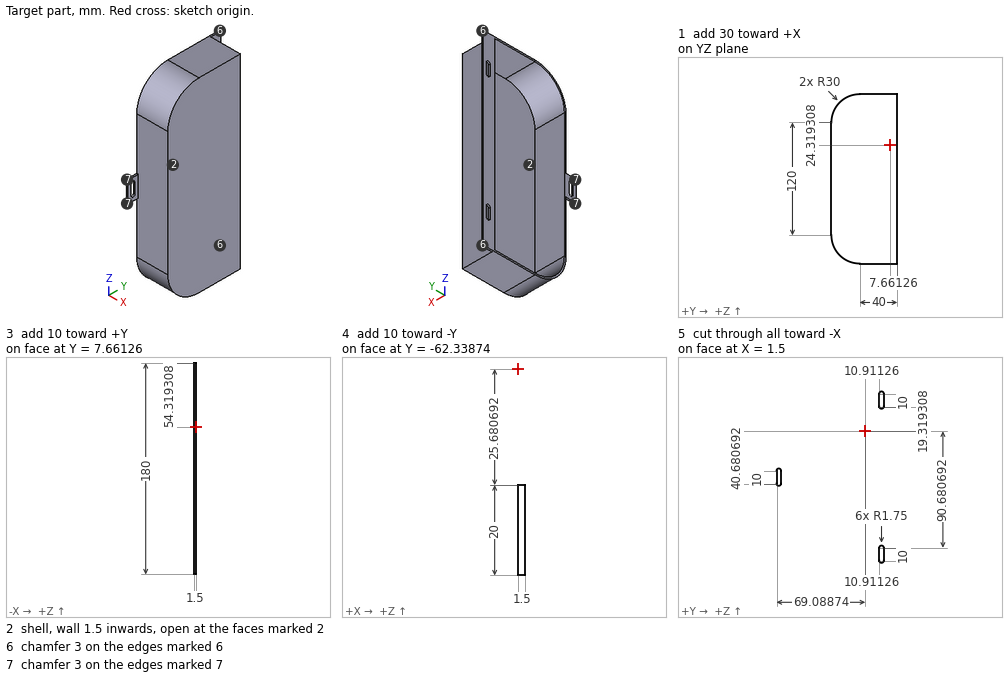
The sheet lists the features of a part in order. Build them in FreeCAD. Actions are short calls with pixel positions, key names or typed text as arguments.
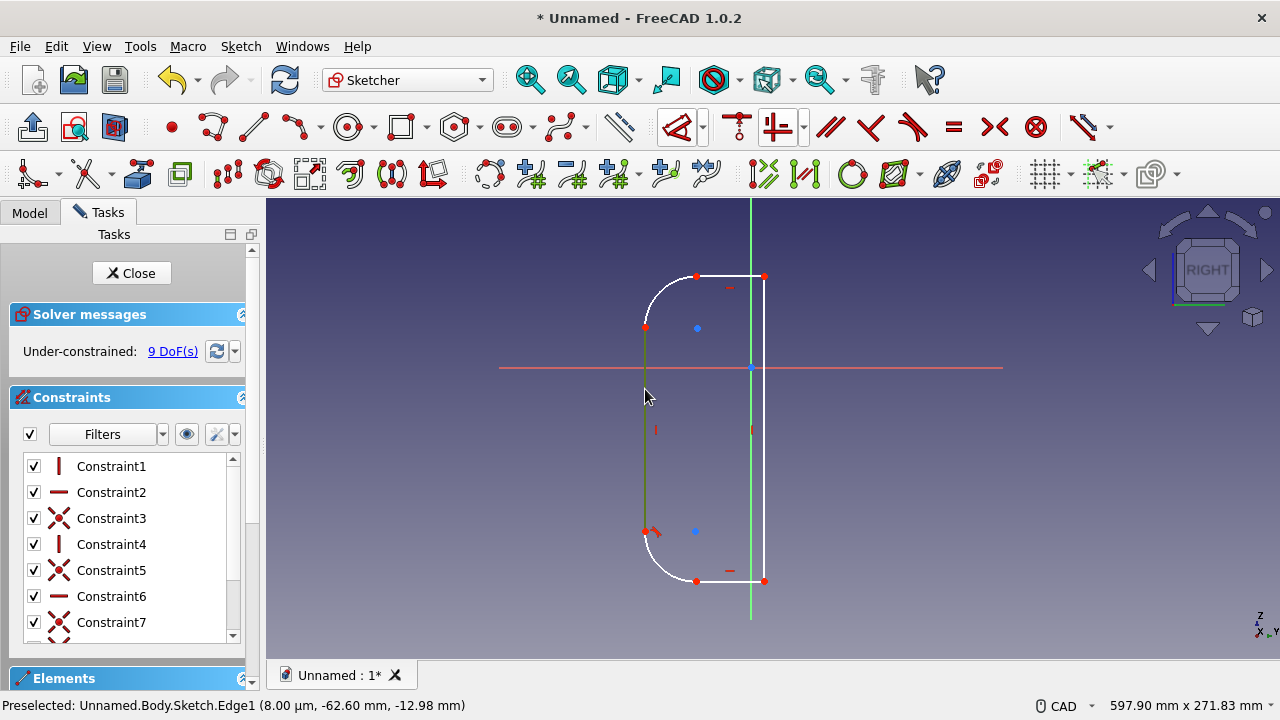
click(673, 282)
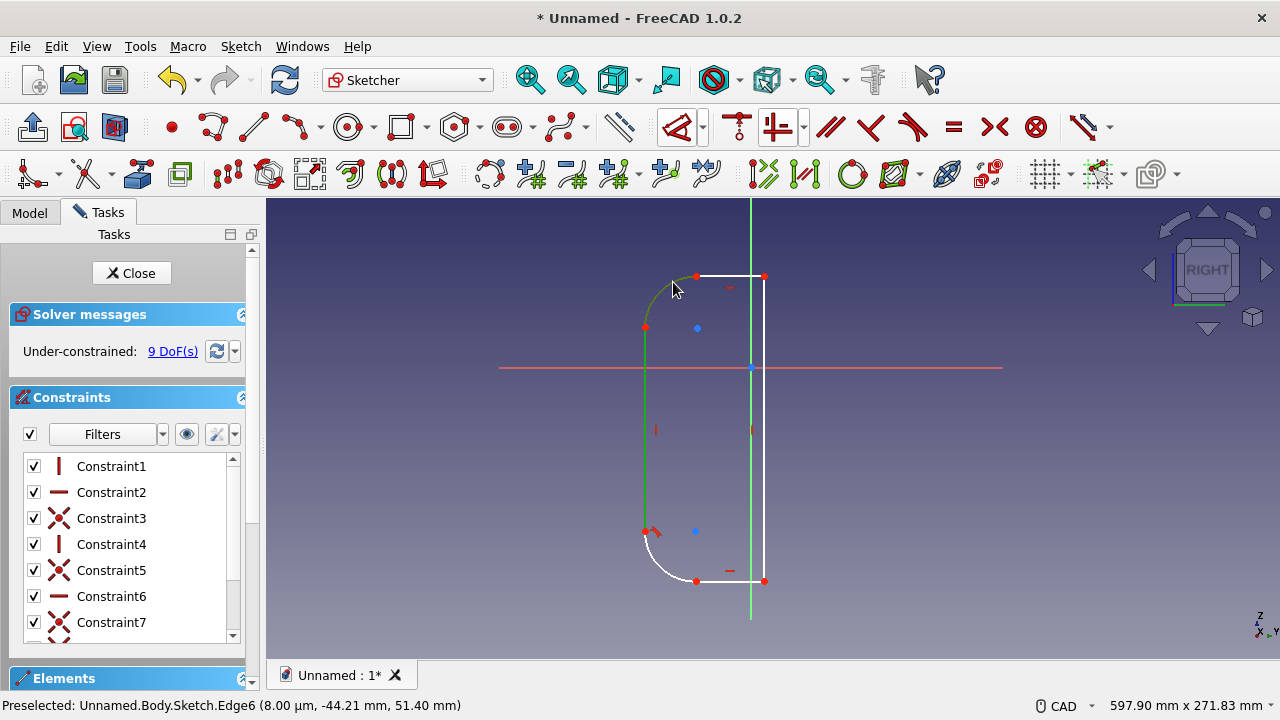
click(913, 128)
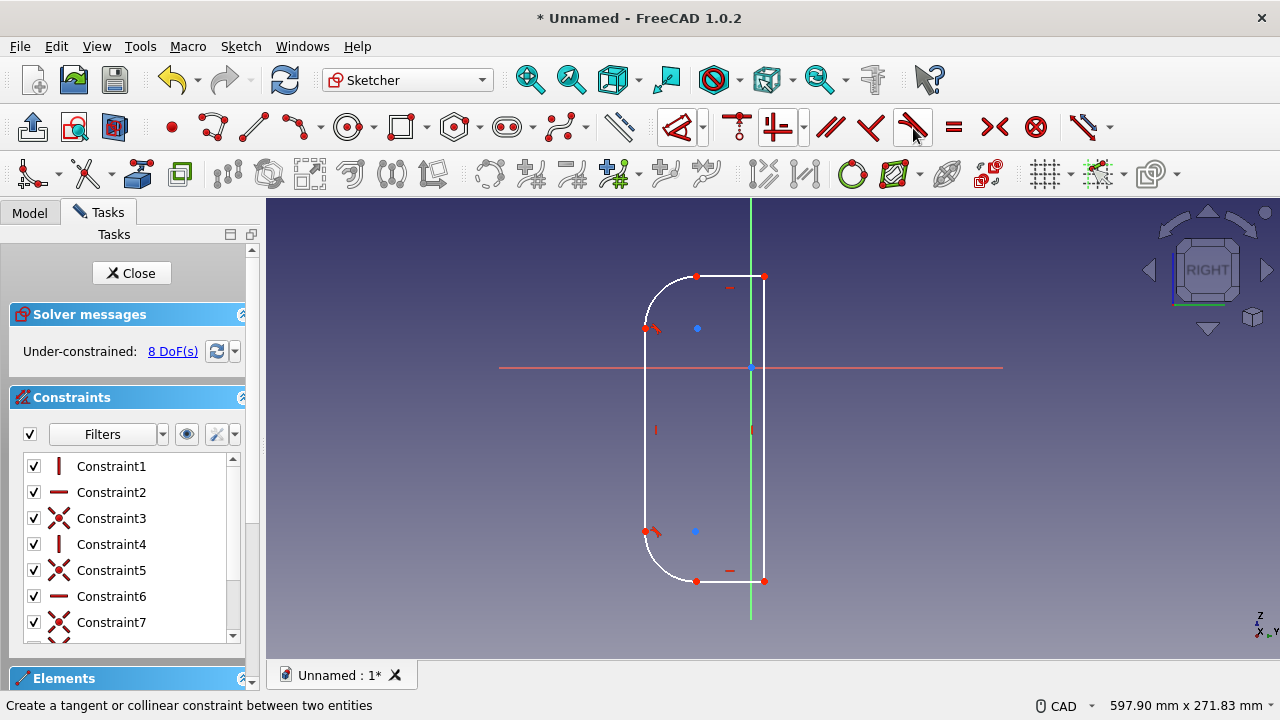
click(716, 582)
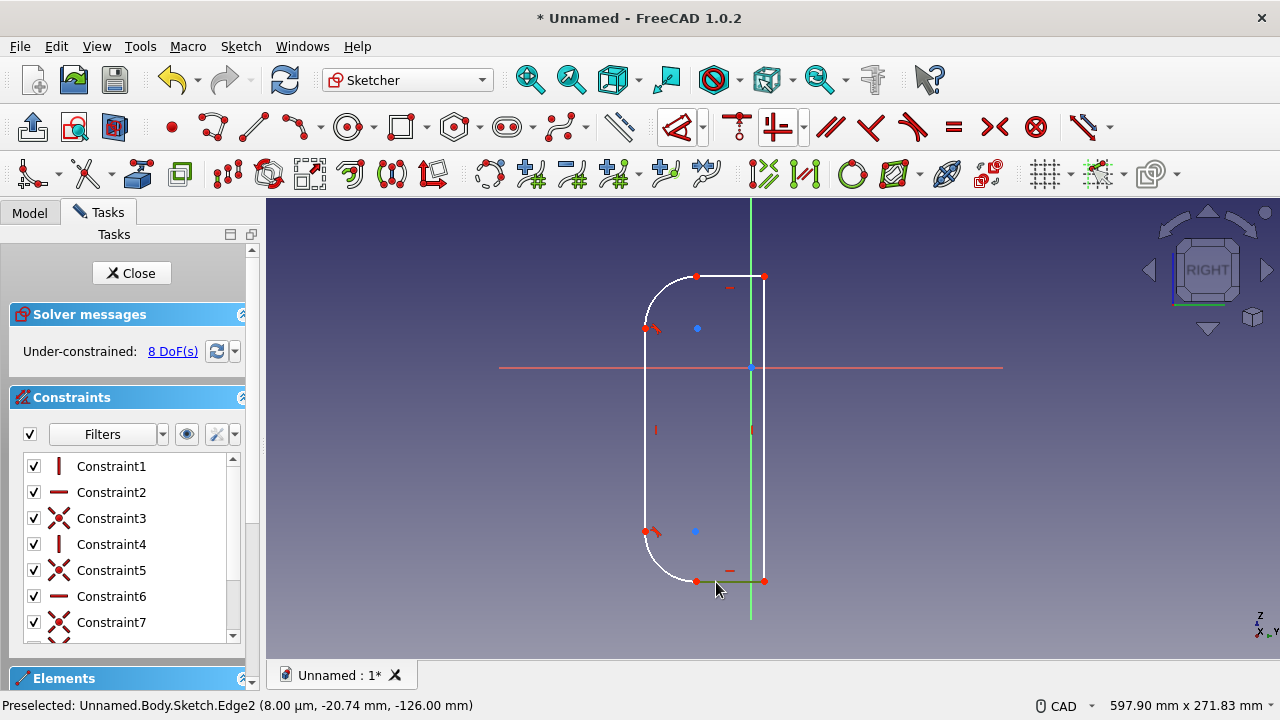
click(651, 554)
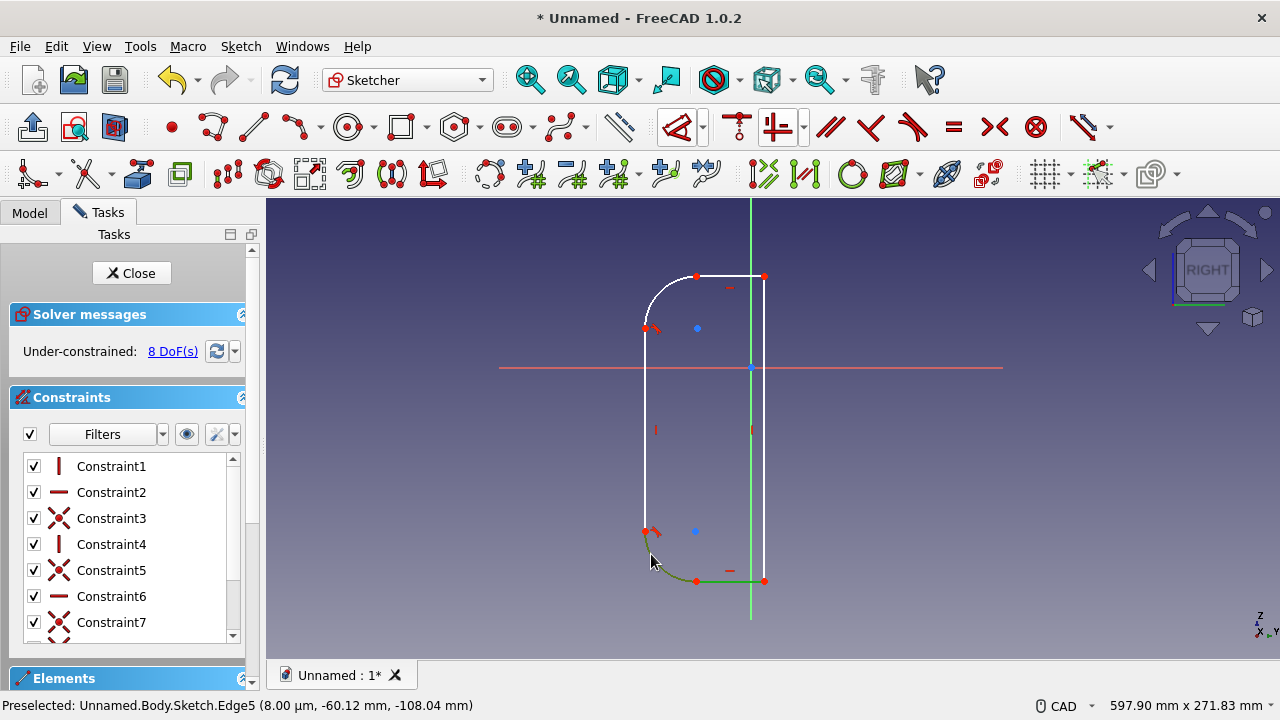
click(913, 128)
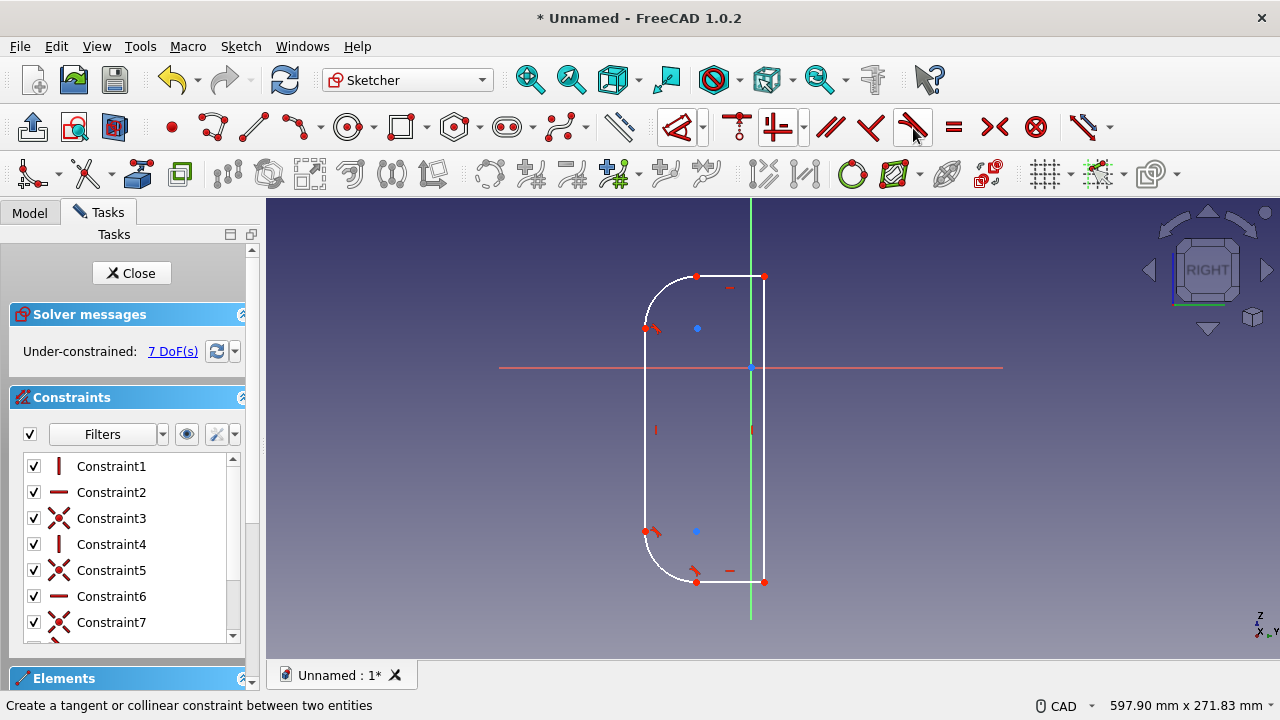
click(717, 276)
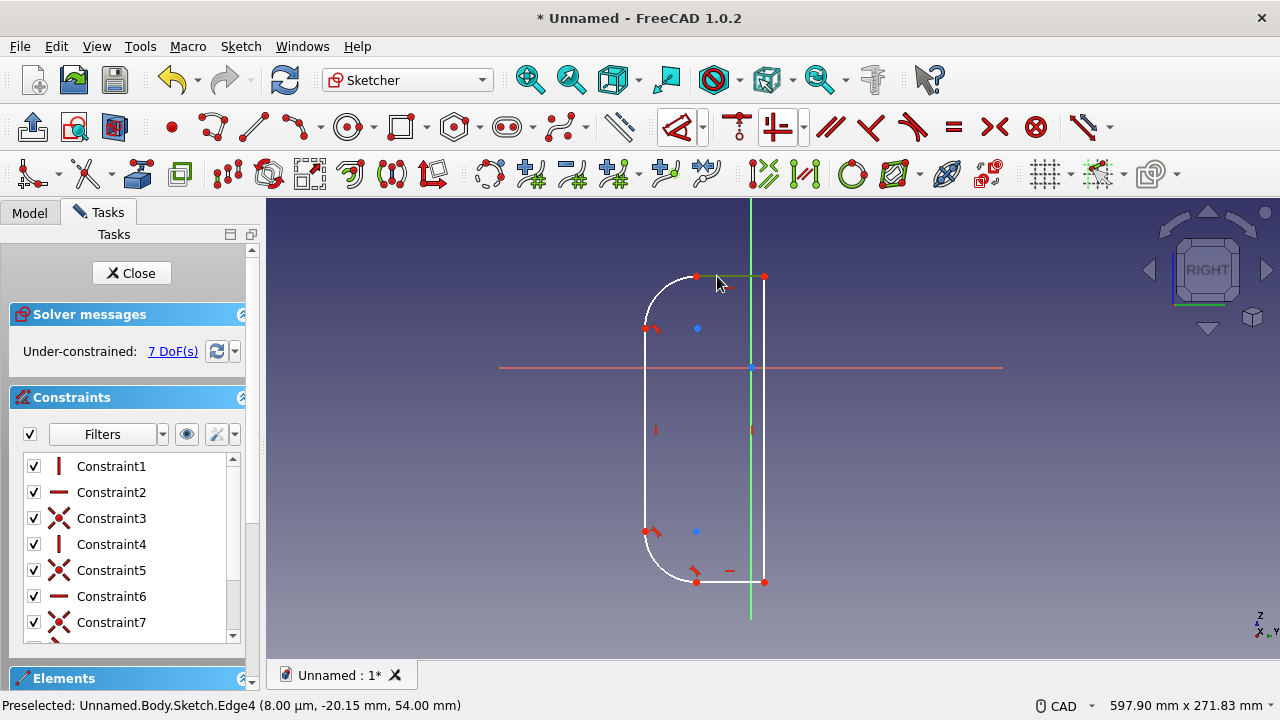
click(673, 282)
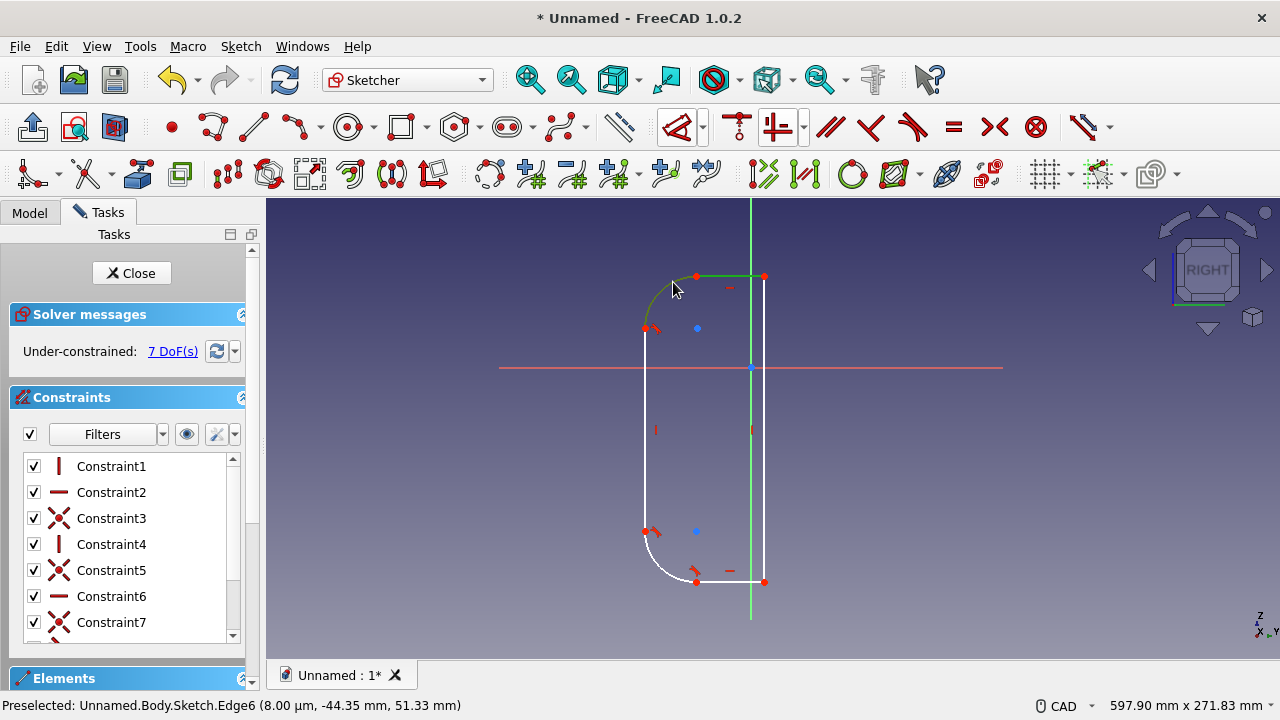
click(913, 128)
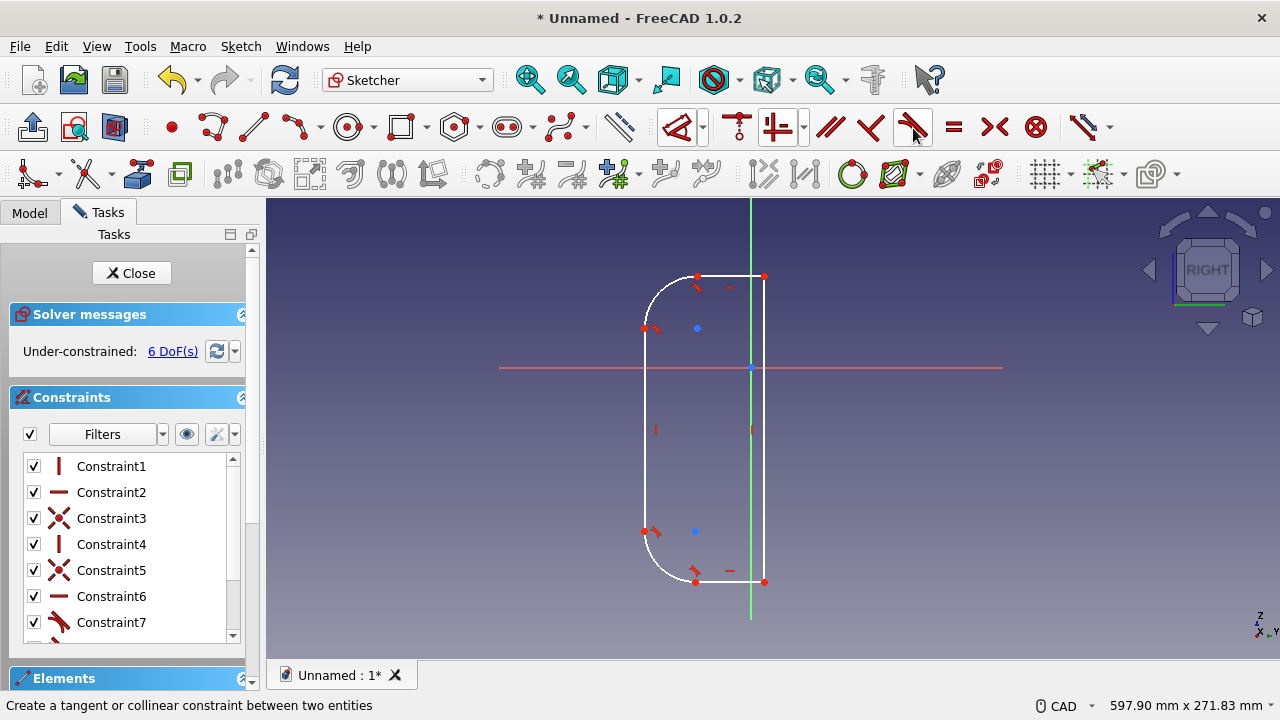
click(650, 554)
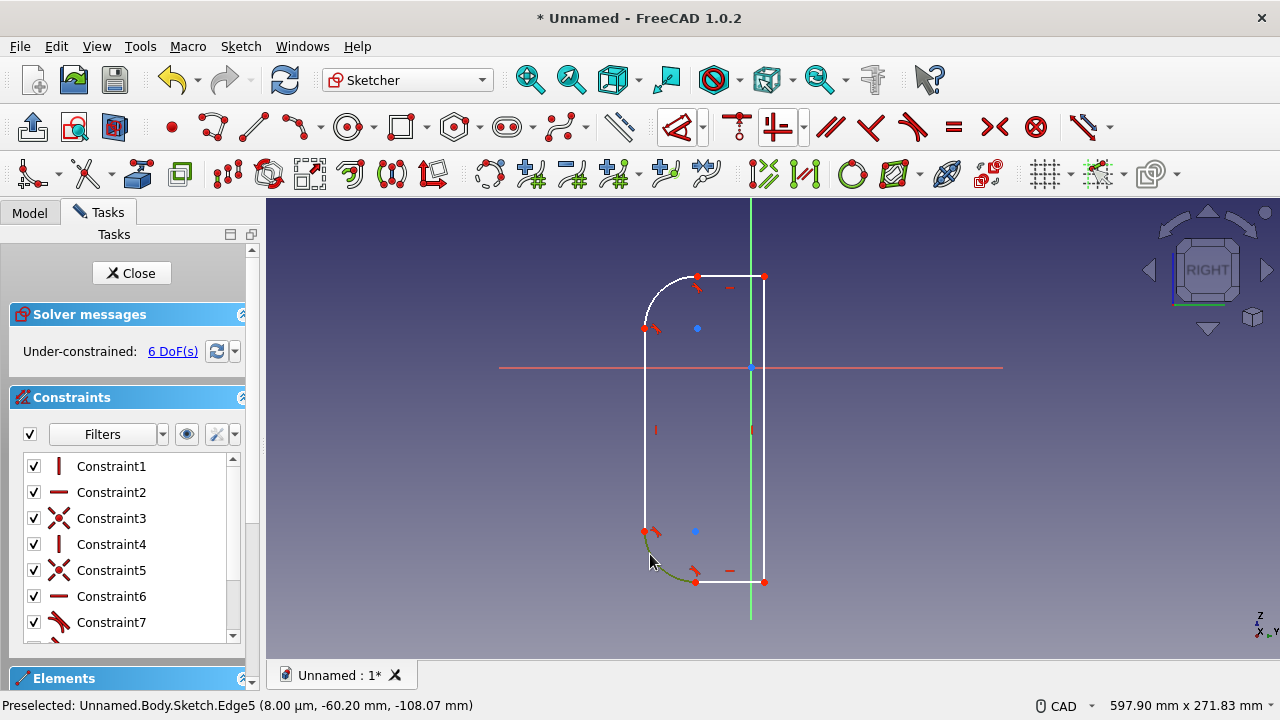
click(673, 282)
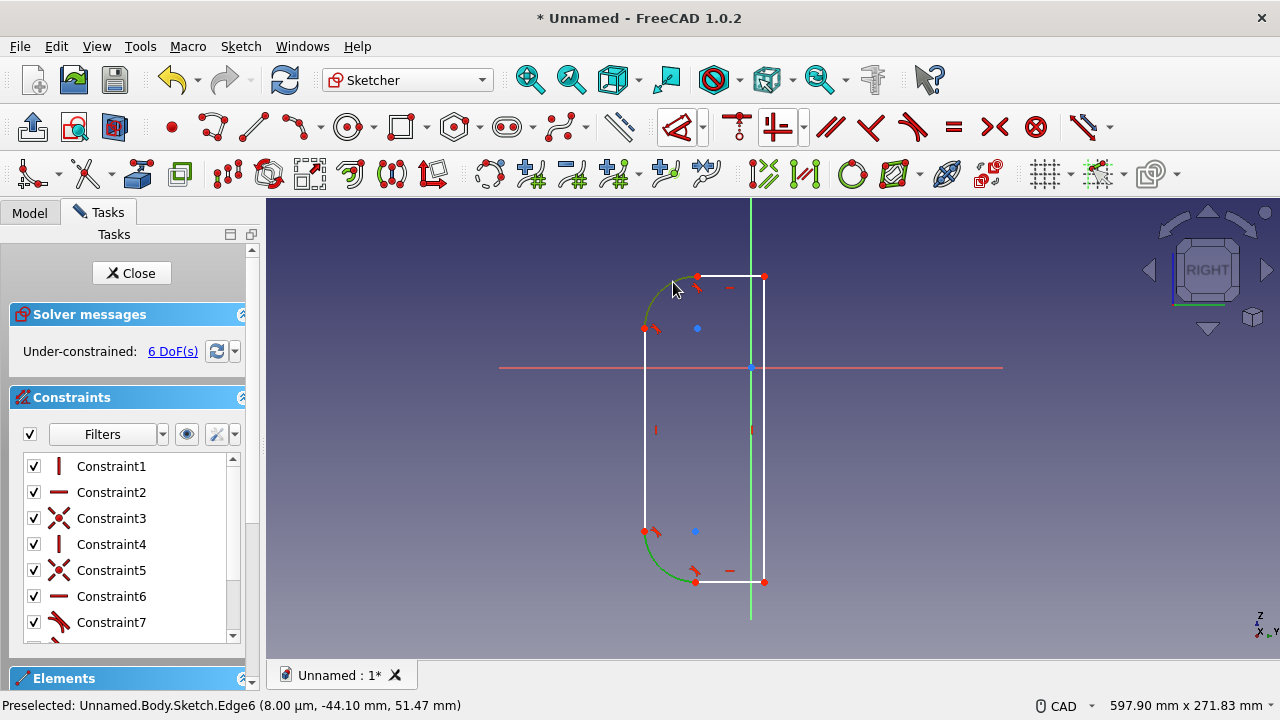
click(954, 128)